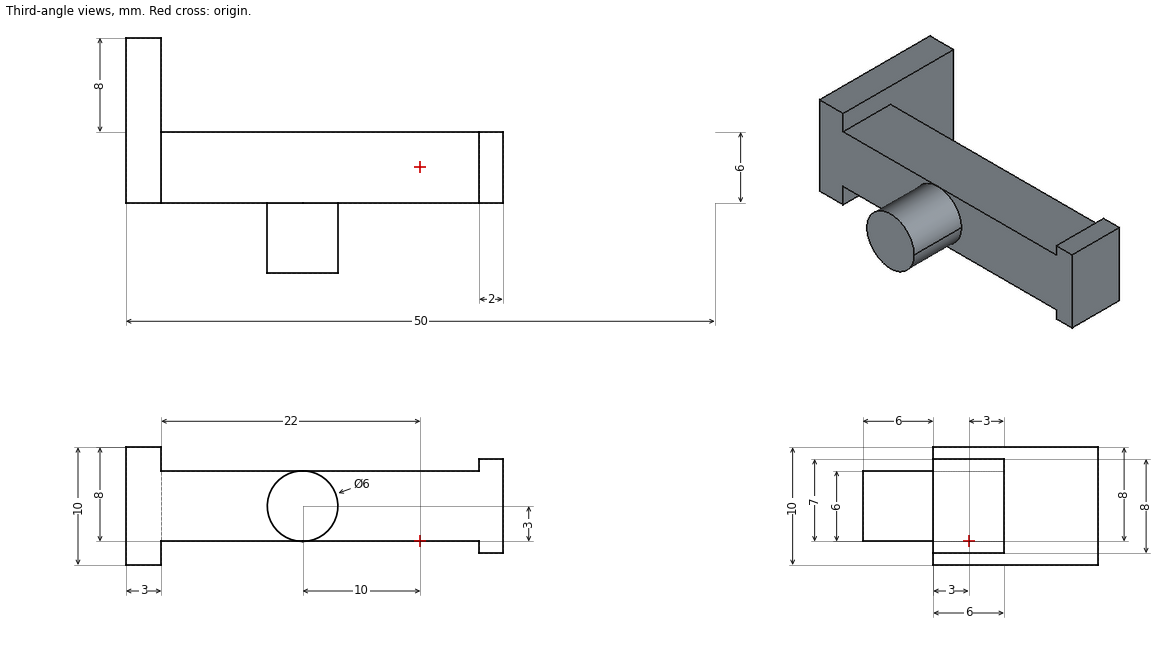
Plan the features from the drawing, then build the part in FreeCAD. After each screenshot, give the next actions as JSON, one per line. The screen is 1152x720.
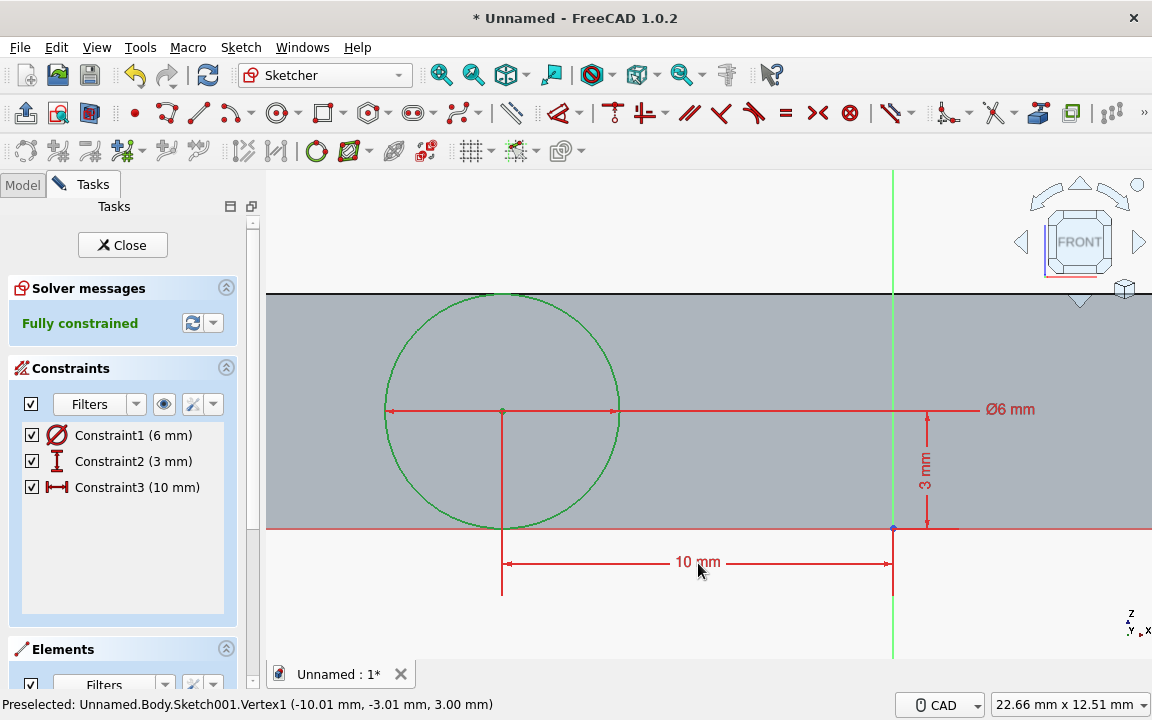
{"action": "left_click", "coordinate": [123, 245]}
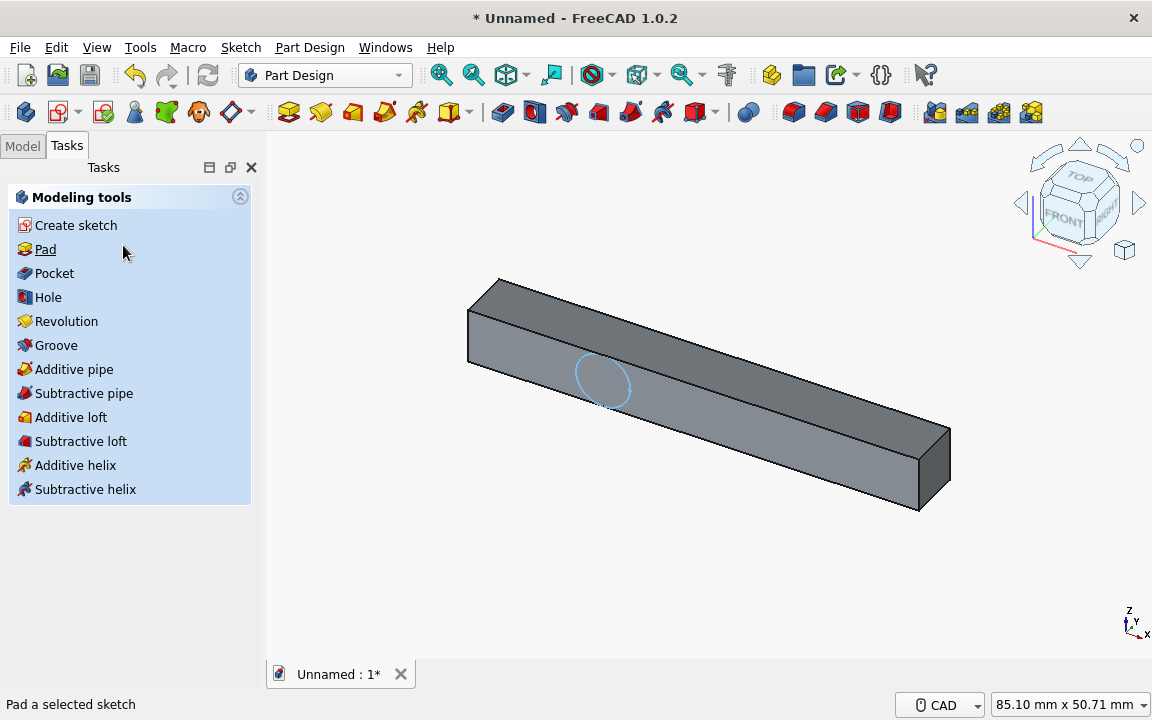
{"action": "left_click", "coordinate": [290, 112]}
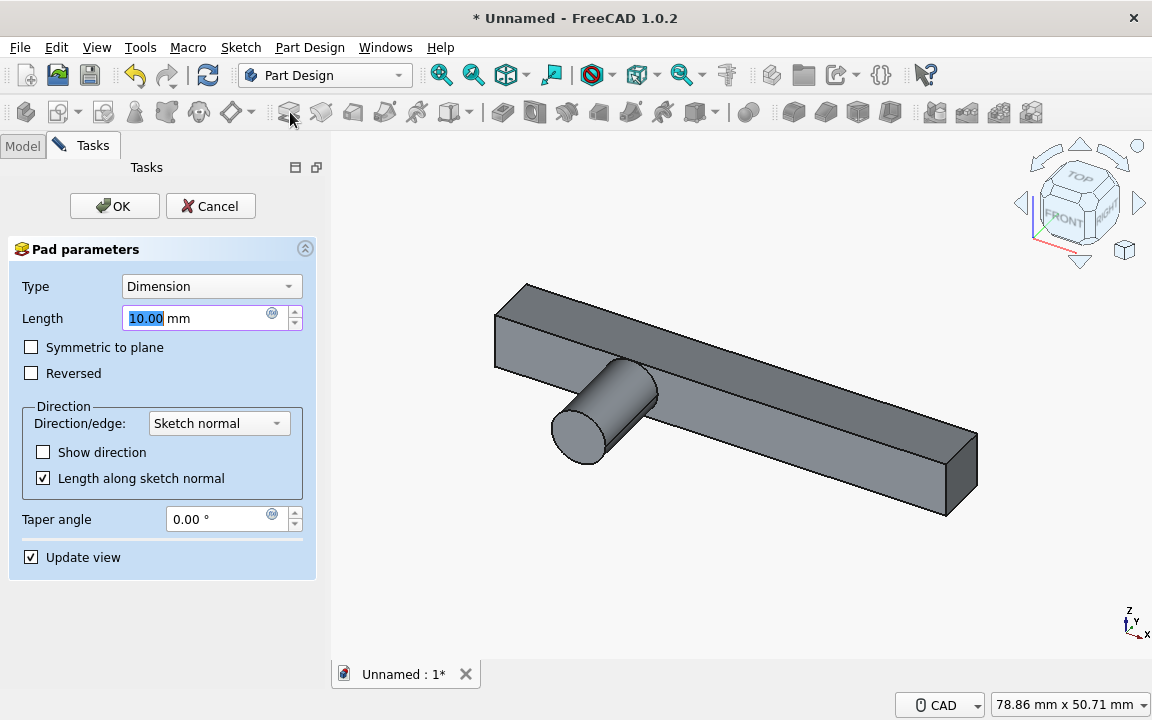
{"action": "type", "text": "6"}
{"action": "key", "text": "Tab"}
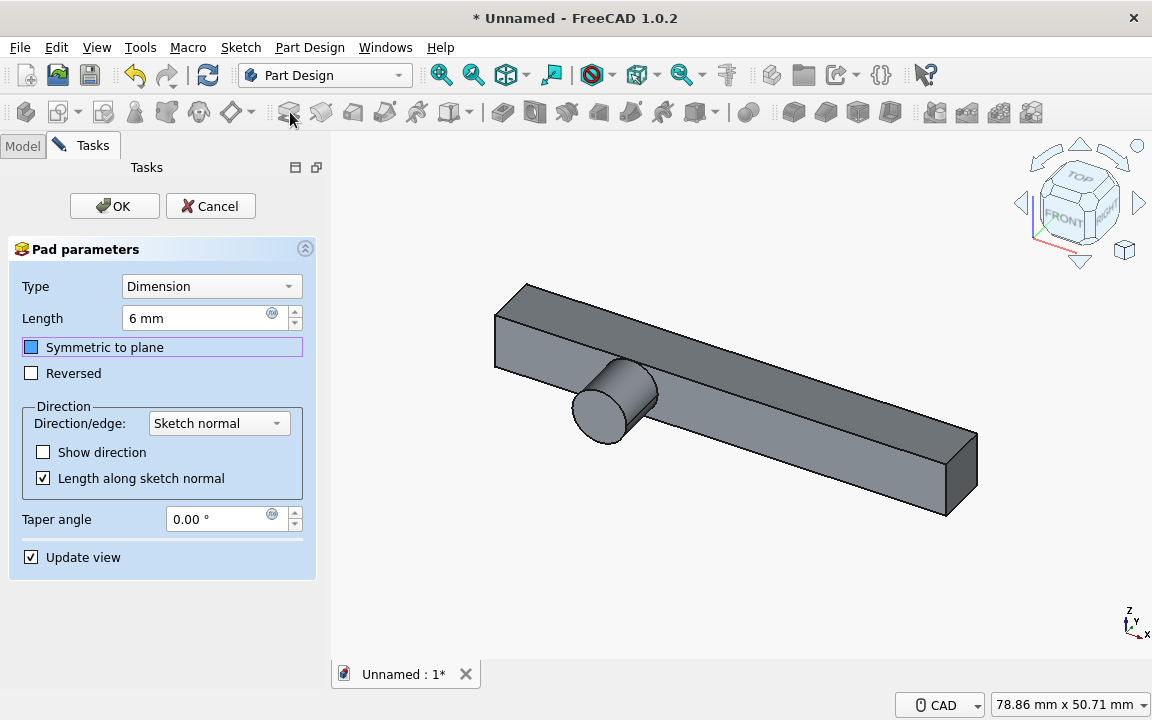
{"action": "left_click", "coordinate": [115, 206]}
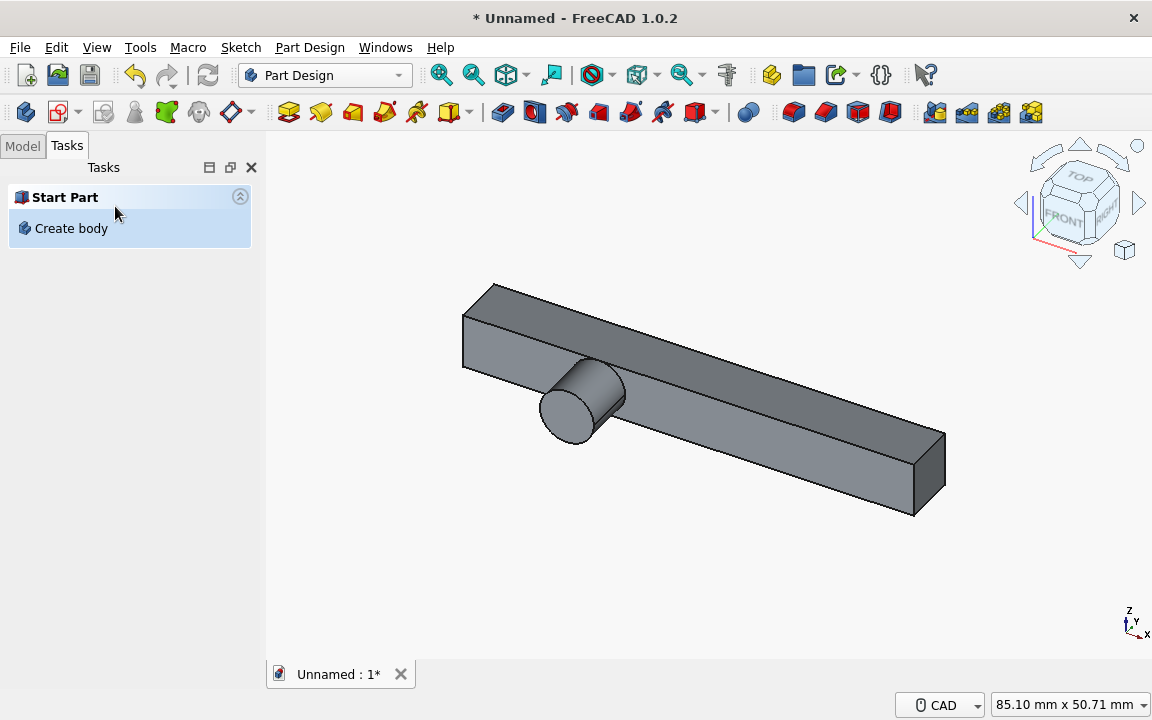
{"action": "key", "text": "6"}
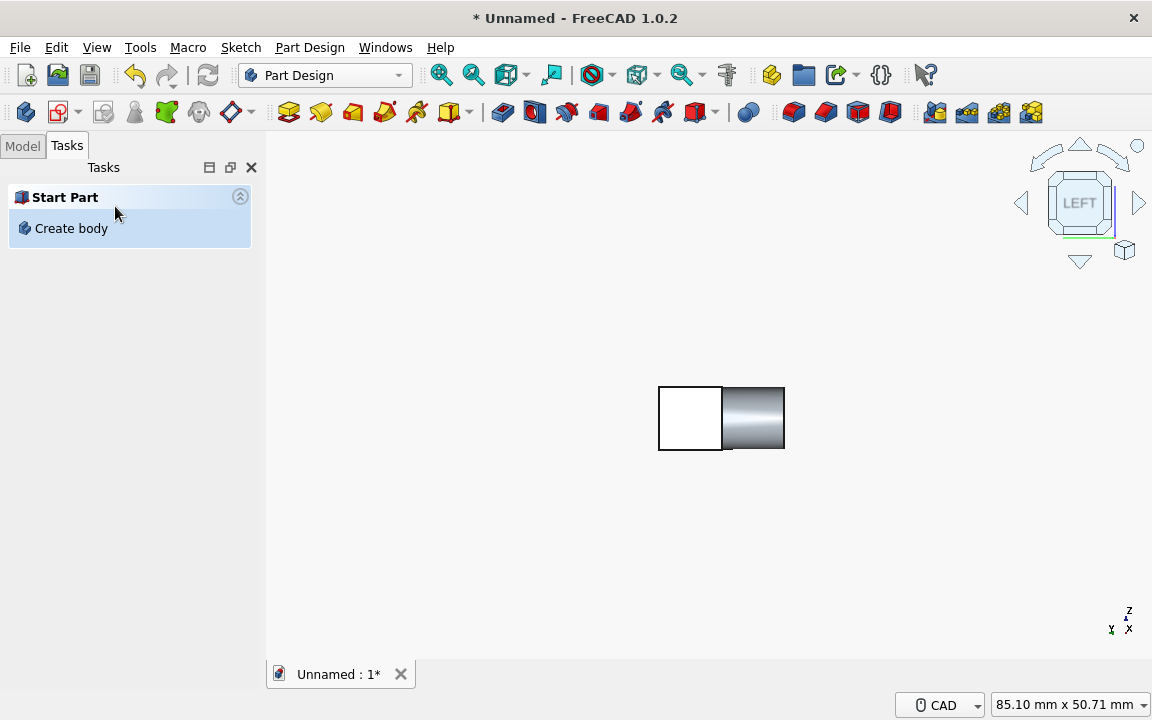
{"action": "left_click", "coordinate": [442, 76]}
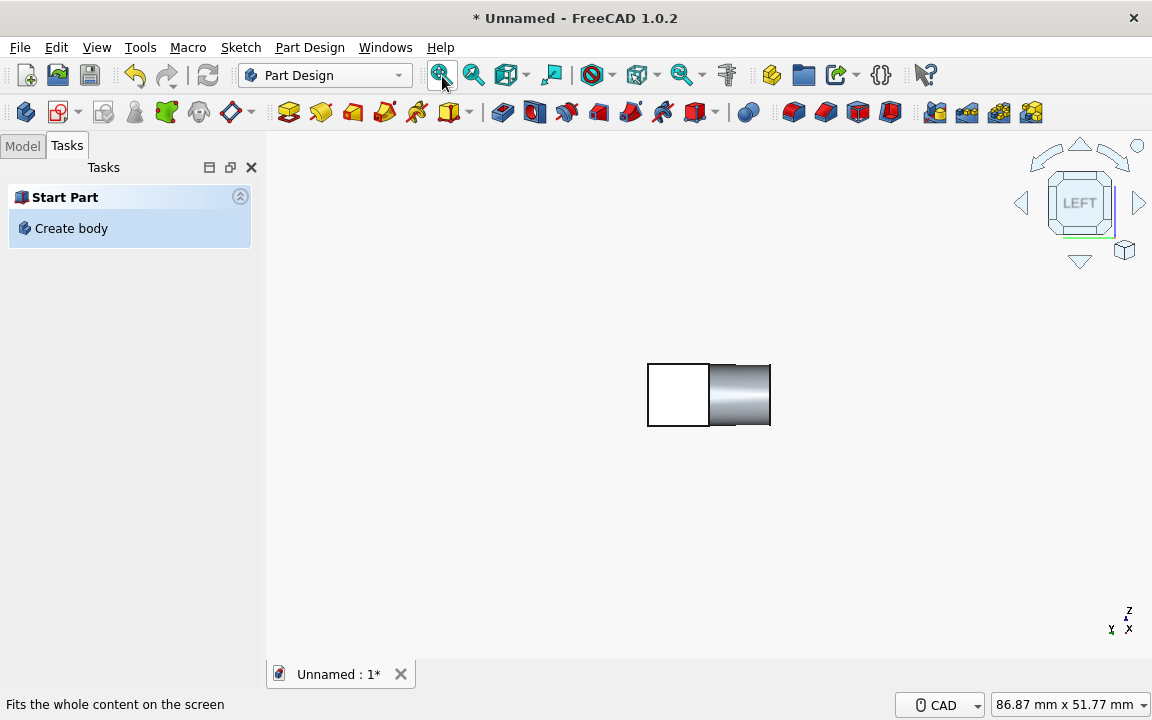
{"action": "left_click", "coordinate": [678, 394]}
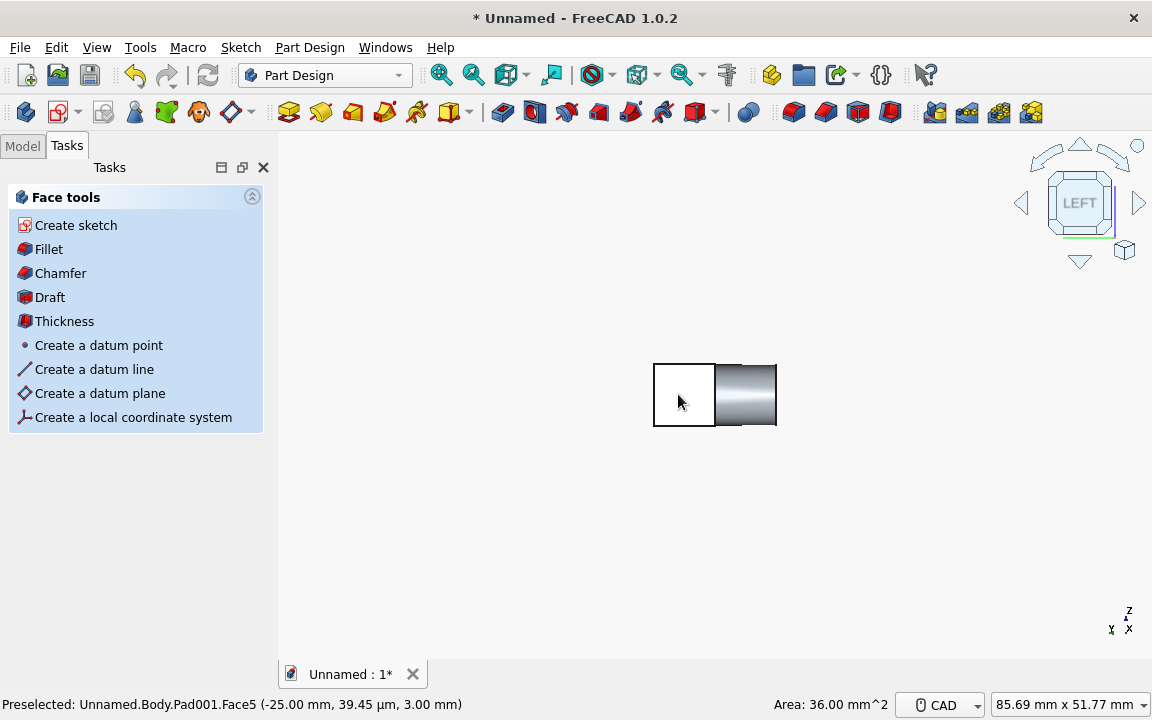
{"action": "left_click", "coordinate": [58, 112]}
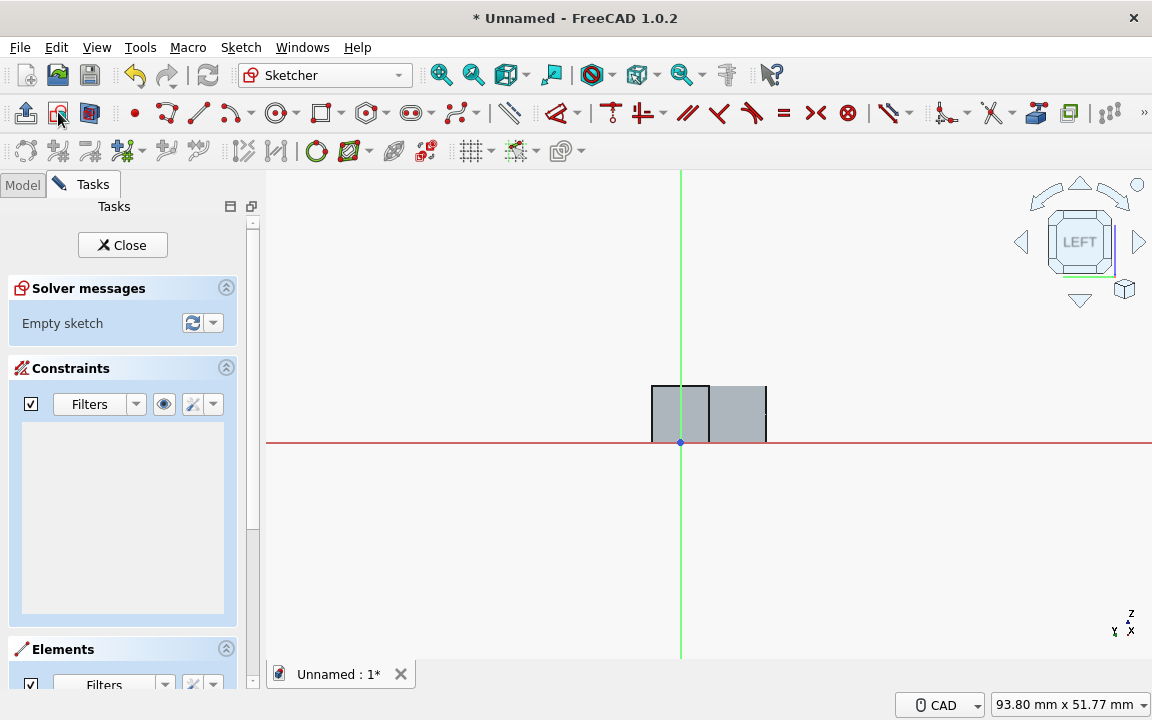
{"action": "scroll", "coordinate": [698, 415], "scroll_direction": "up", "scroll_amount": 6}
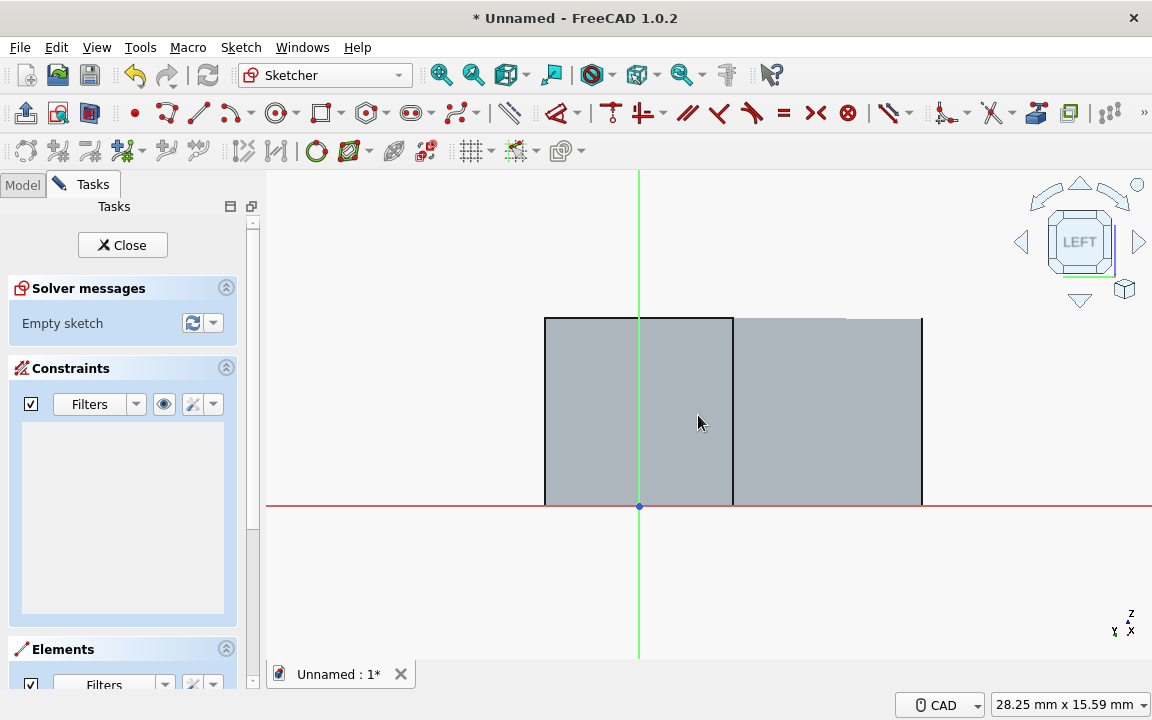
{"action": "left_click", "coordinate": [322, 114]}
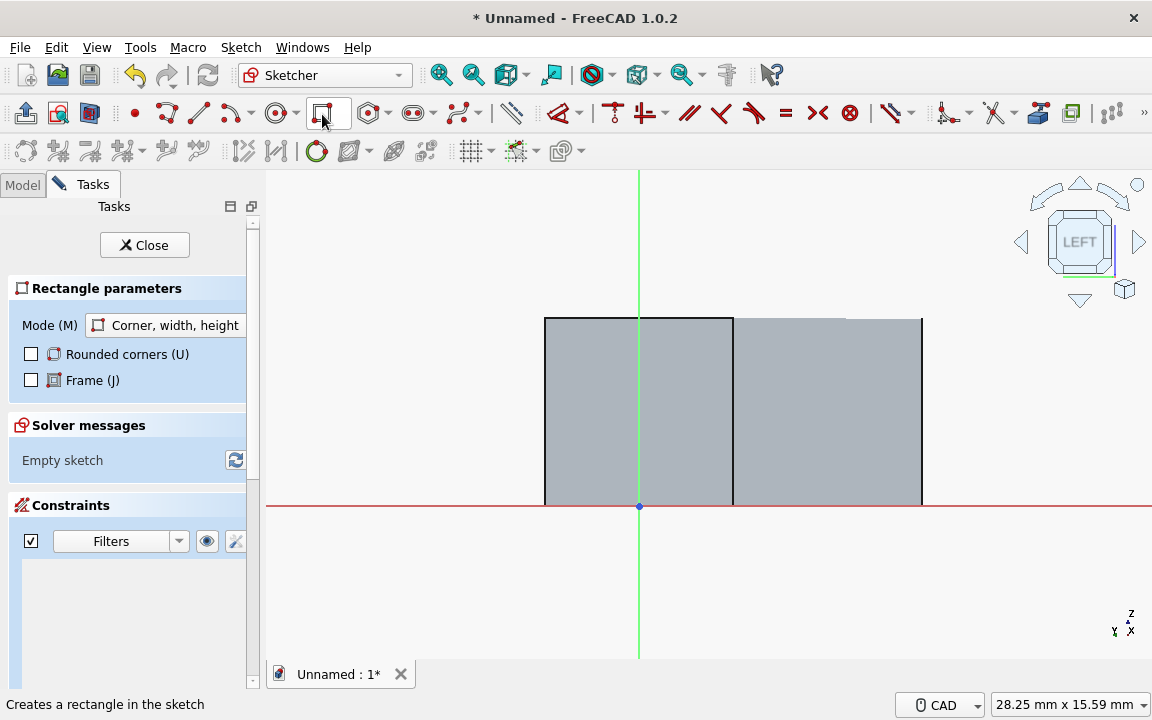
{"action": "left_click", "coordinate": [545, 255]}
{"action": "mouse_move", "coordinate": [733, 569]}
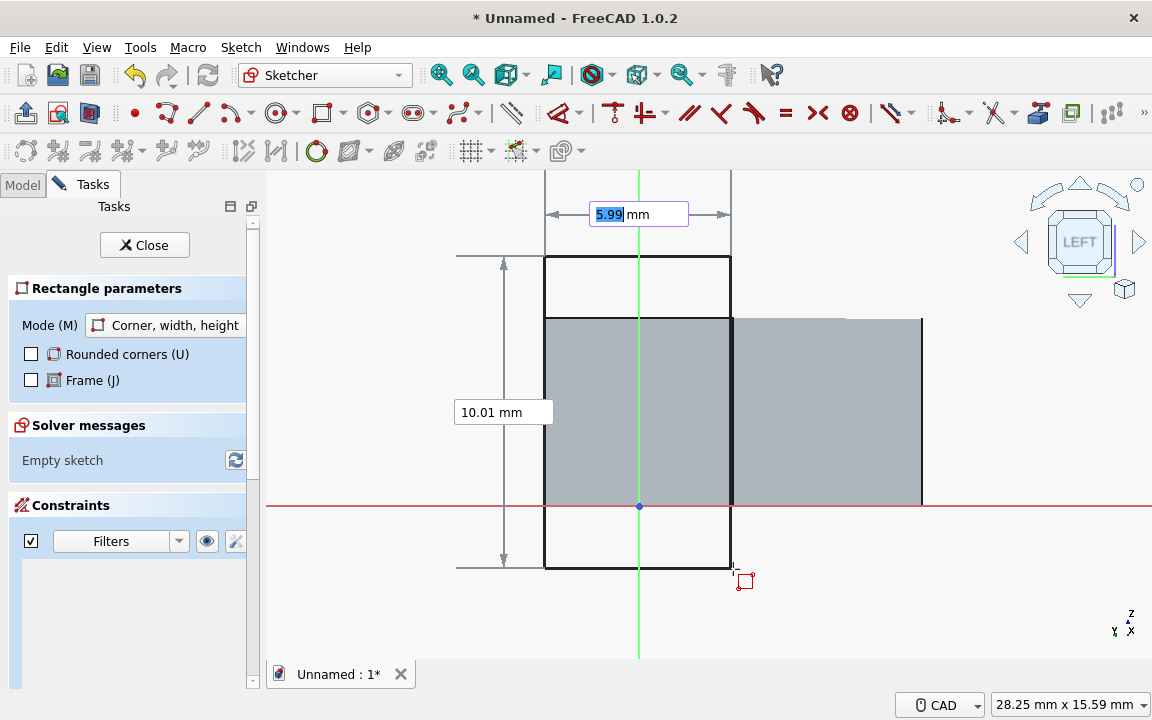
{"action": "type", "text": "6"}
{"action": "key", "text": "Tab"}
{"action": "type", "text": "10"}
{"action": "key", "text": "Return"}
{"action": "key", "text": "Escape"}